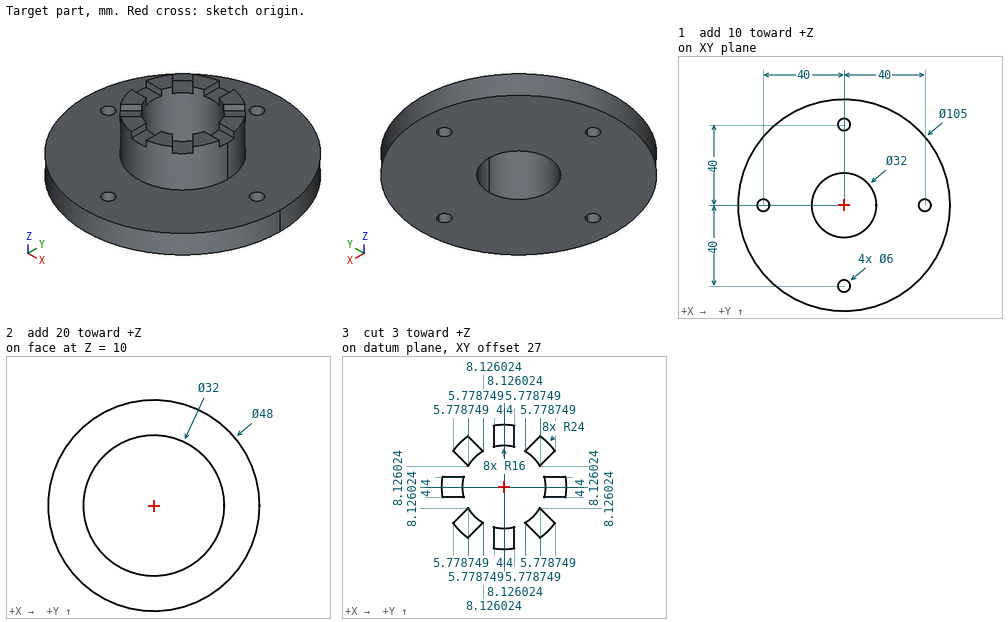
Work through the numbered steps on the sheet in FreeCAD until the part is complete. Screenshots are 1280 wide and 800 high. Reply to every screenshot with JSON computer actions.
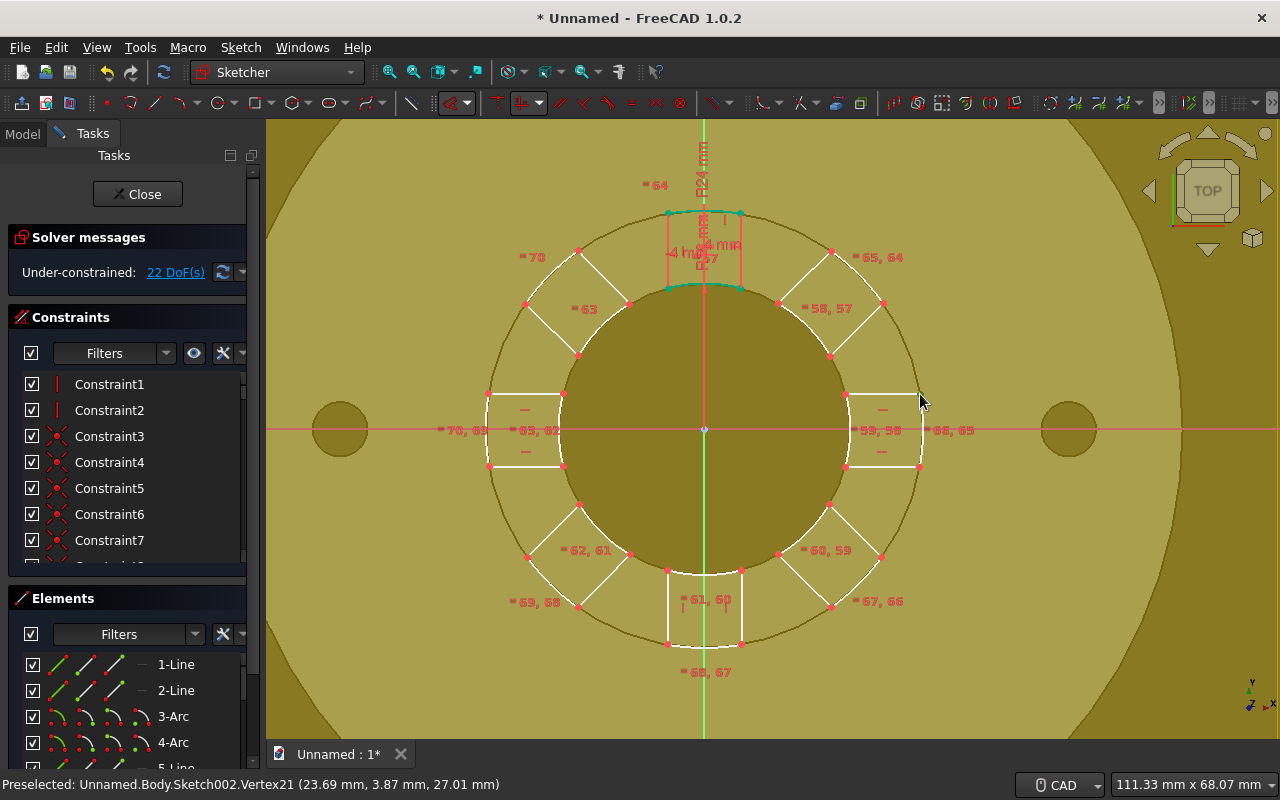
{"action": "left_click", "coordinate": [470, 104]}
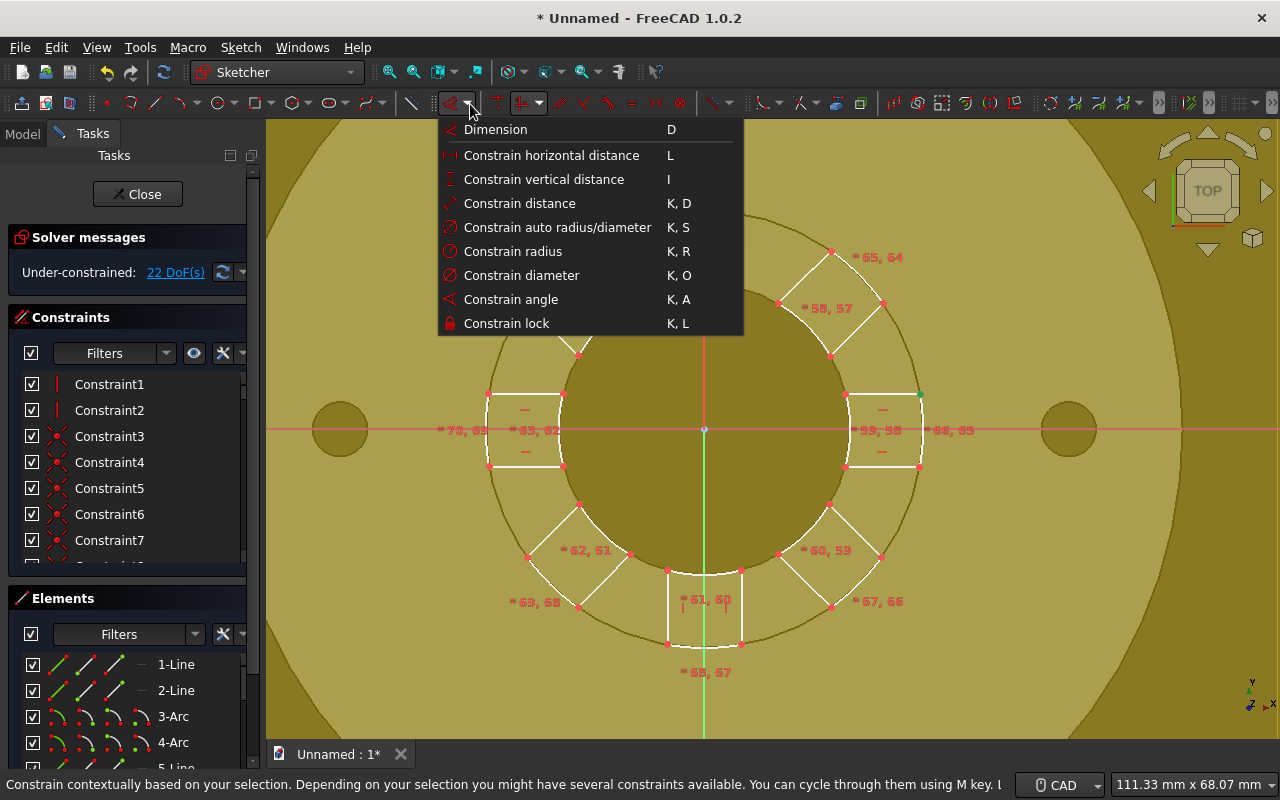
{"action": "left_click", "coordinate": [591, 179]}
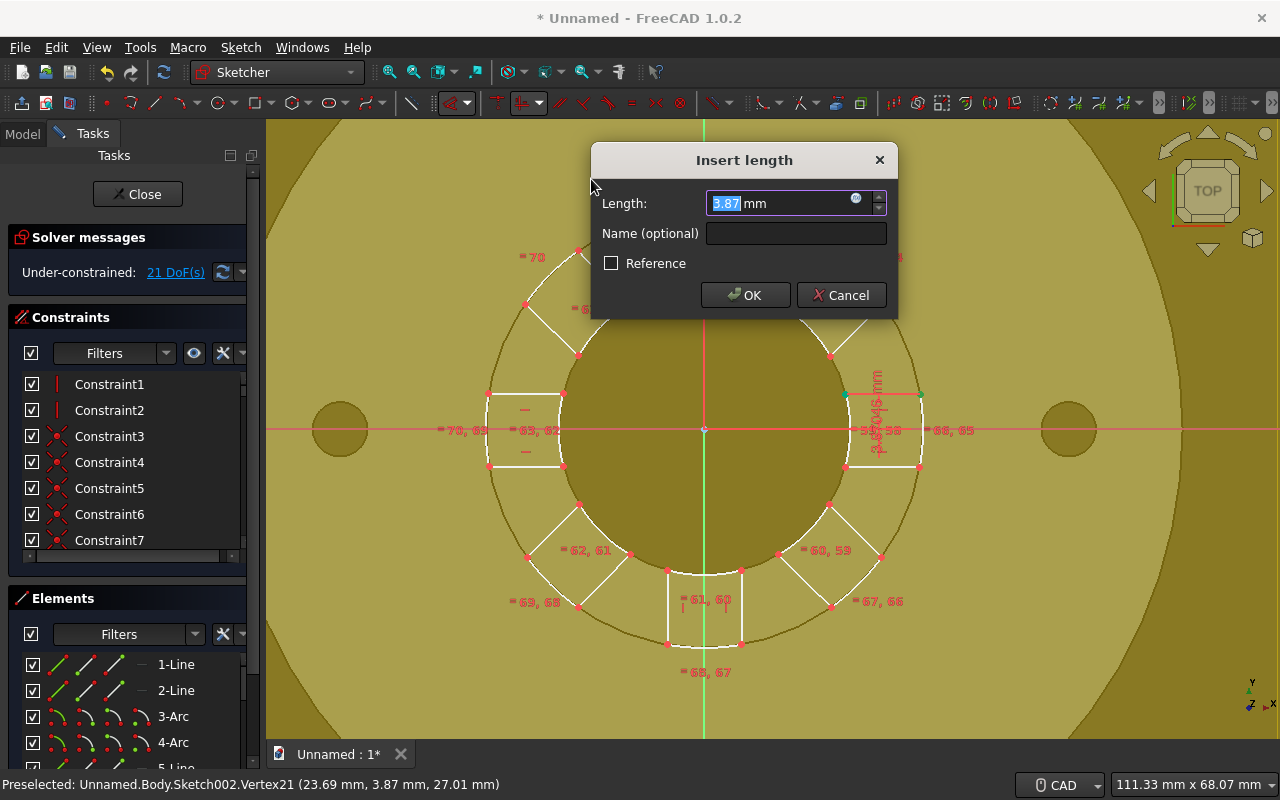
{"action": "type", "text": "4"}
{"action": "key", "text": "Return"}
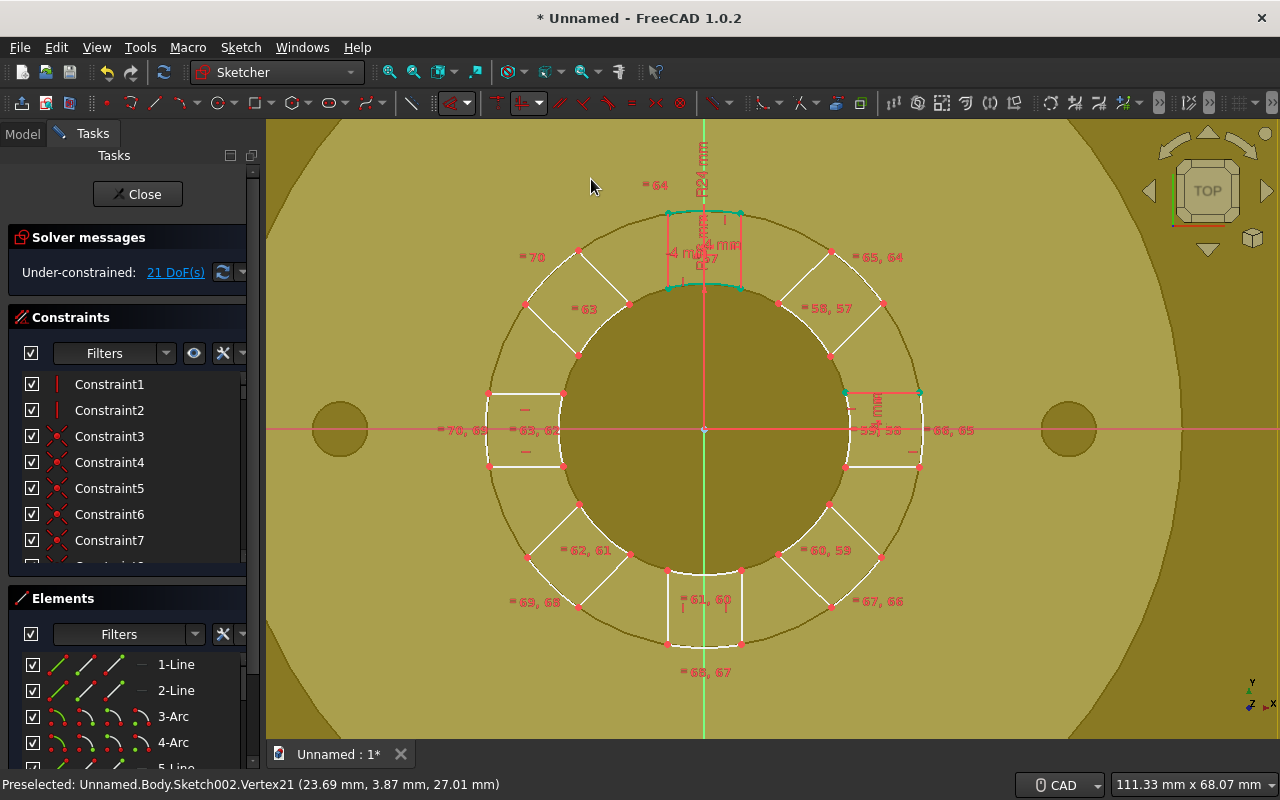
{"action": "left_click", "coordinate": [845, 467]}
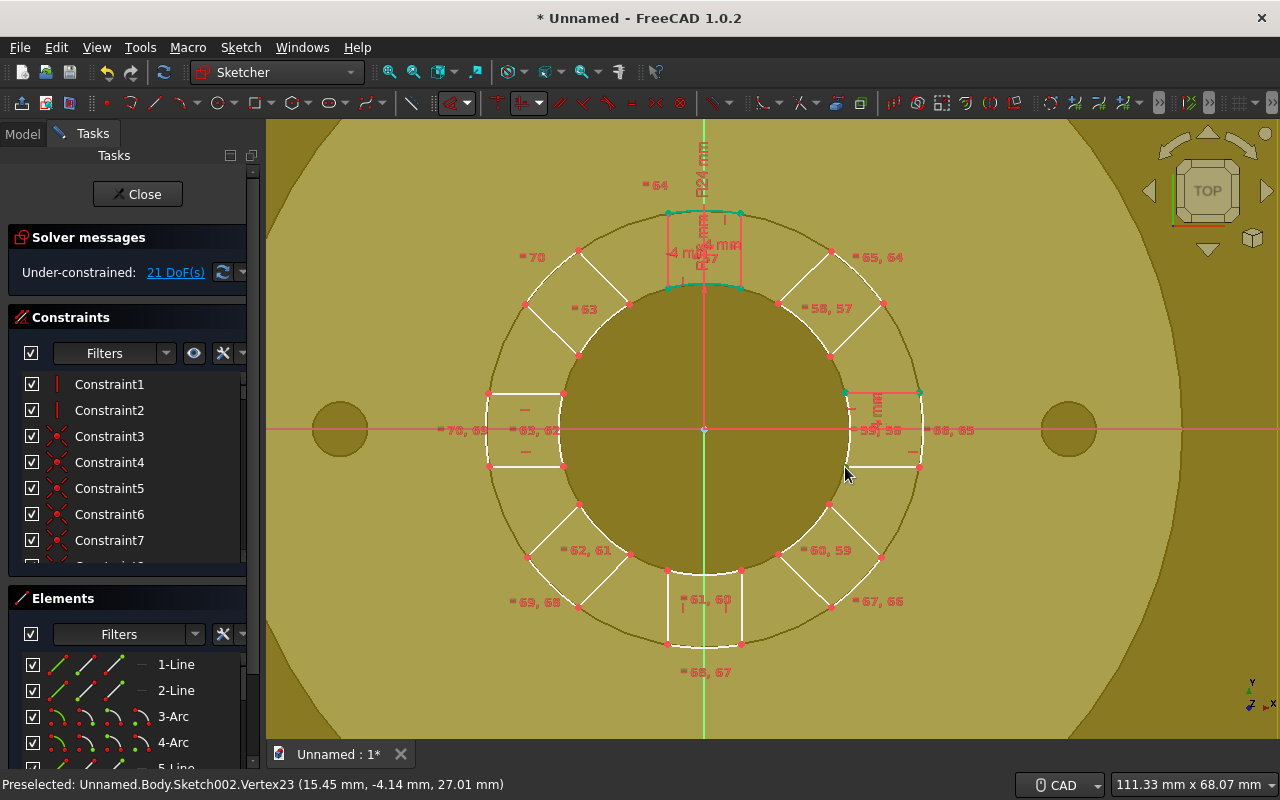
{"action": "key", "text": "i"}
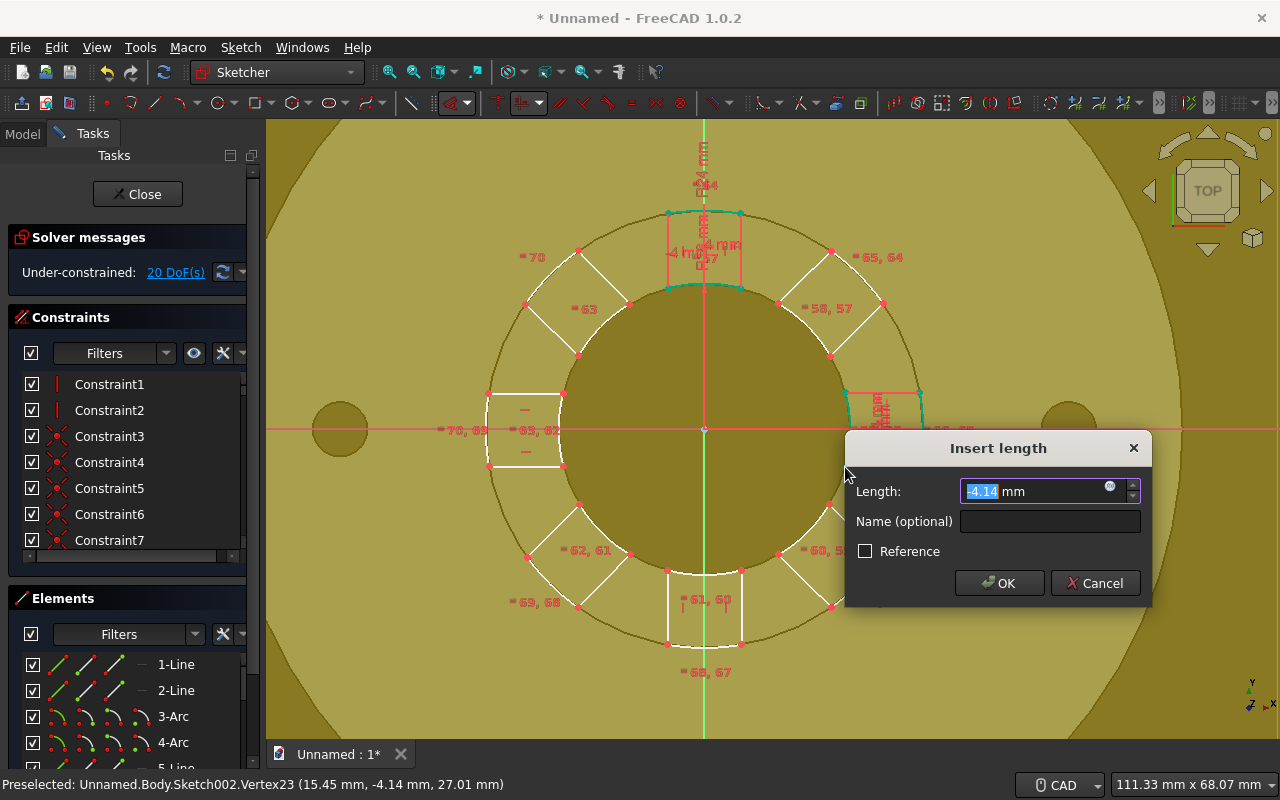
{"action": "type", "text": "-4"}
{"action": "key", "text": "Return"}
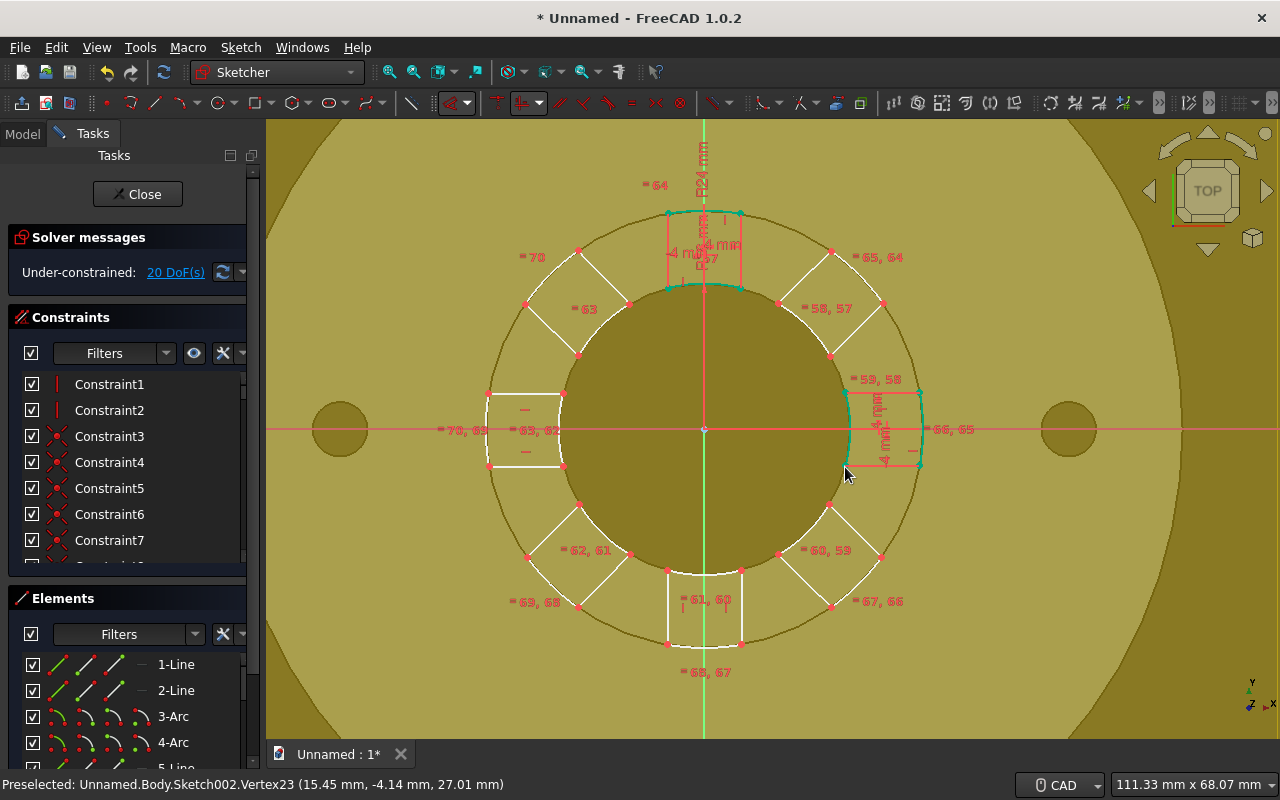
{"action": "left_click", "coordinate": [742, 645]}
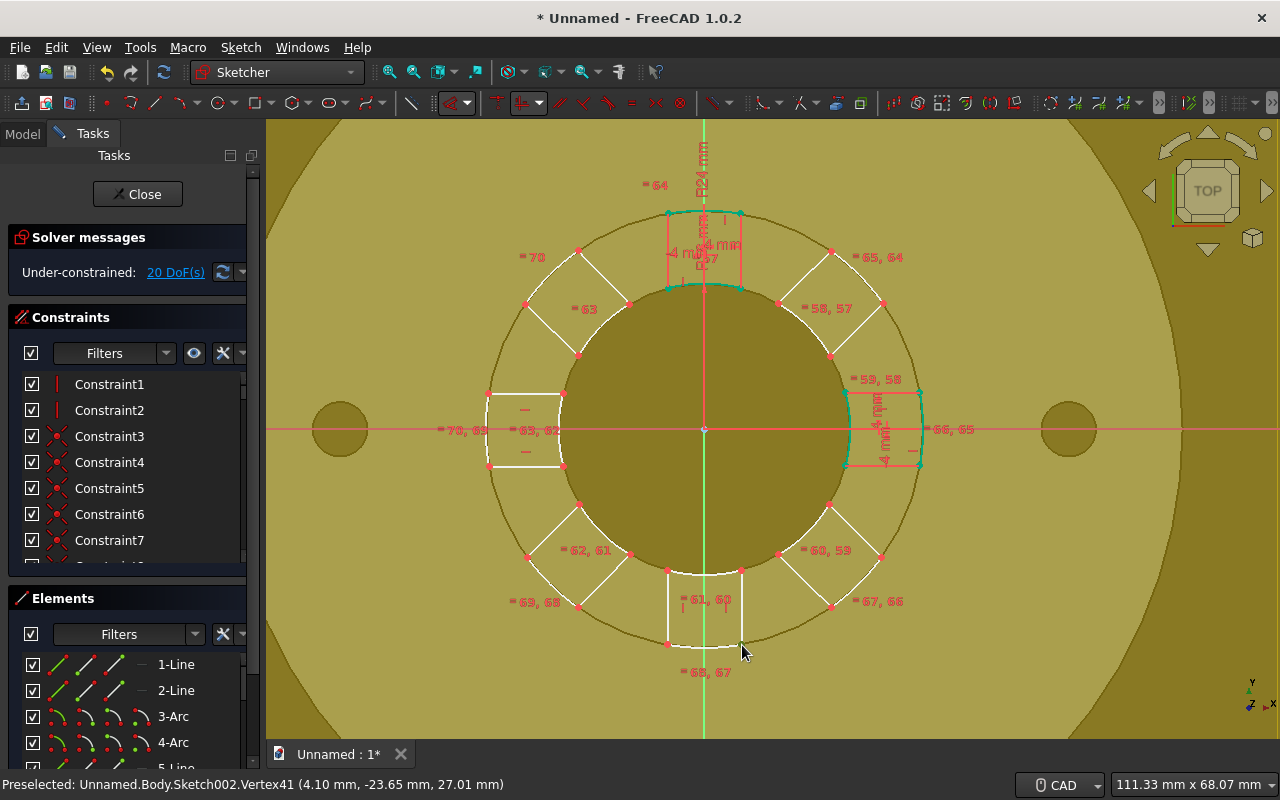
{"action": "left_click", "coordinate": [470, 104]}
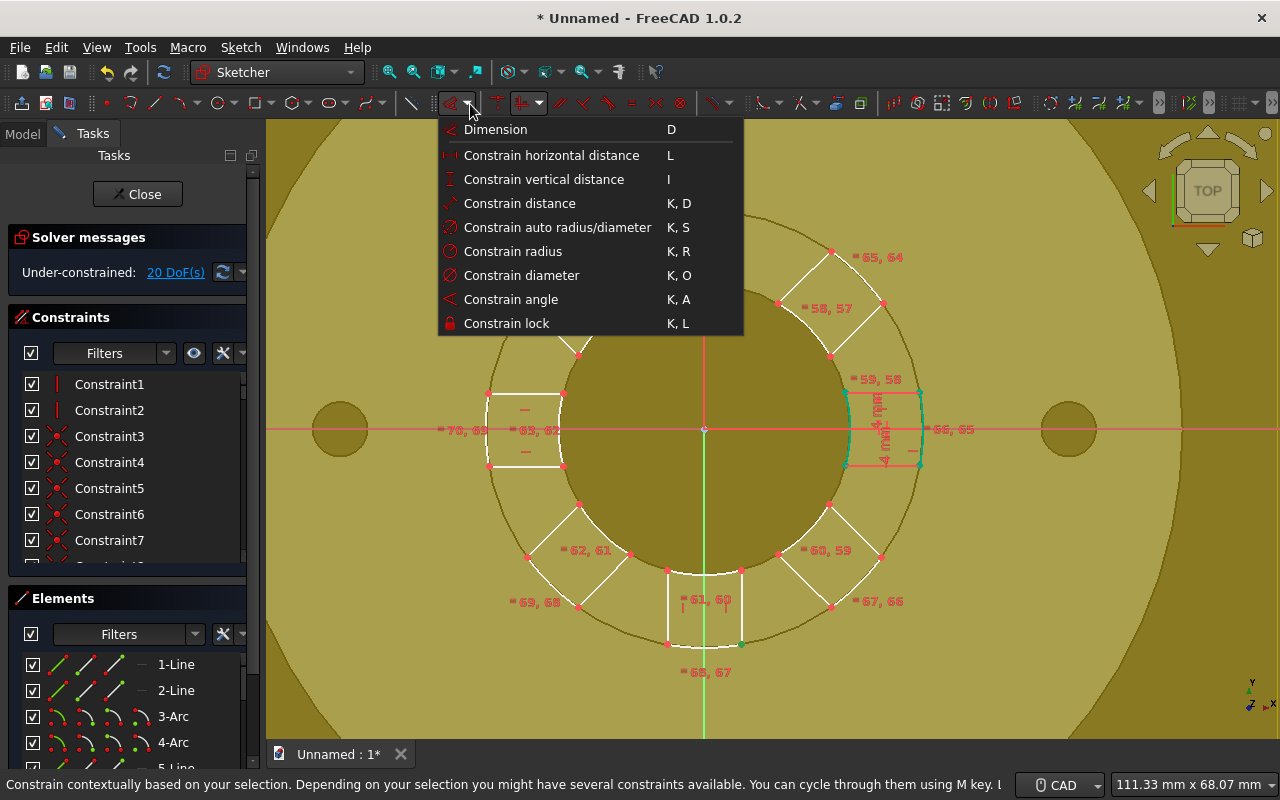
{"action": "left_click", "coordinate": [591, 155]}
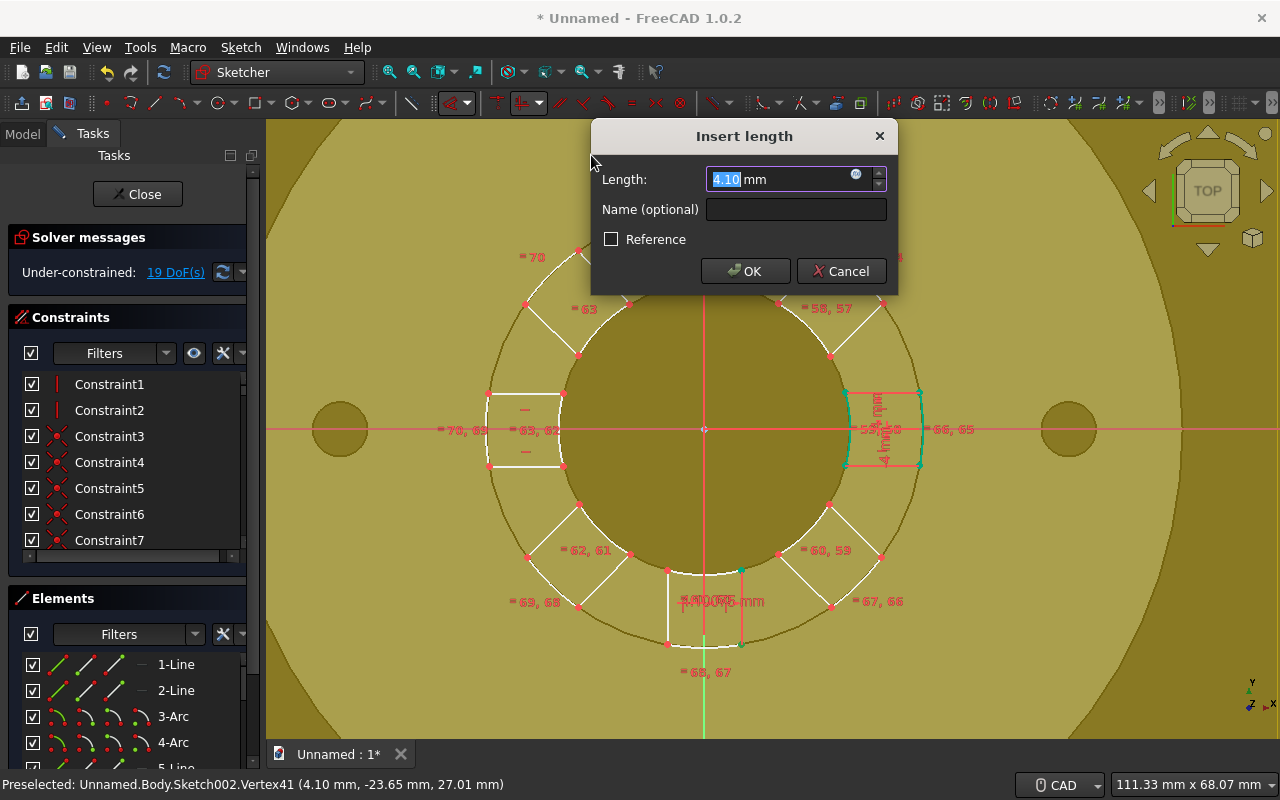
{"action": "type", "text": "4"}
{"action": "key", "text": "Return"}